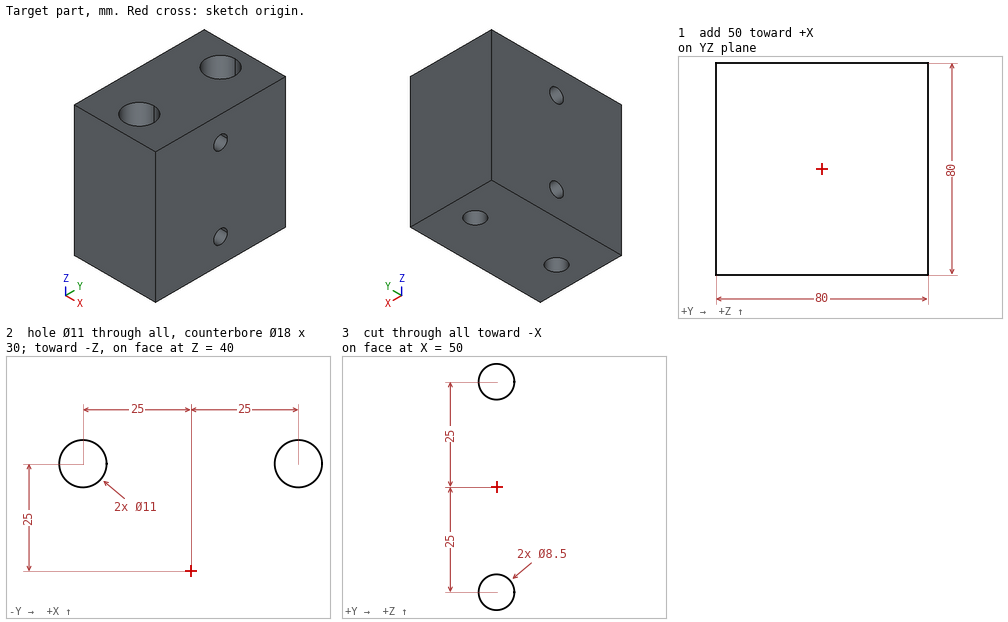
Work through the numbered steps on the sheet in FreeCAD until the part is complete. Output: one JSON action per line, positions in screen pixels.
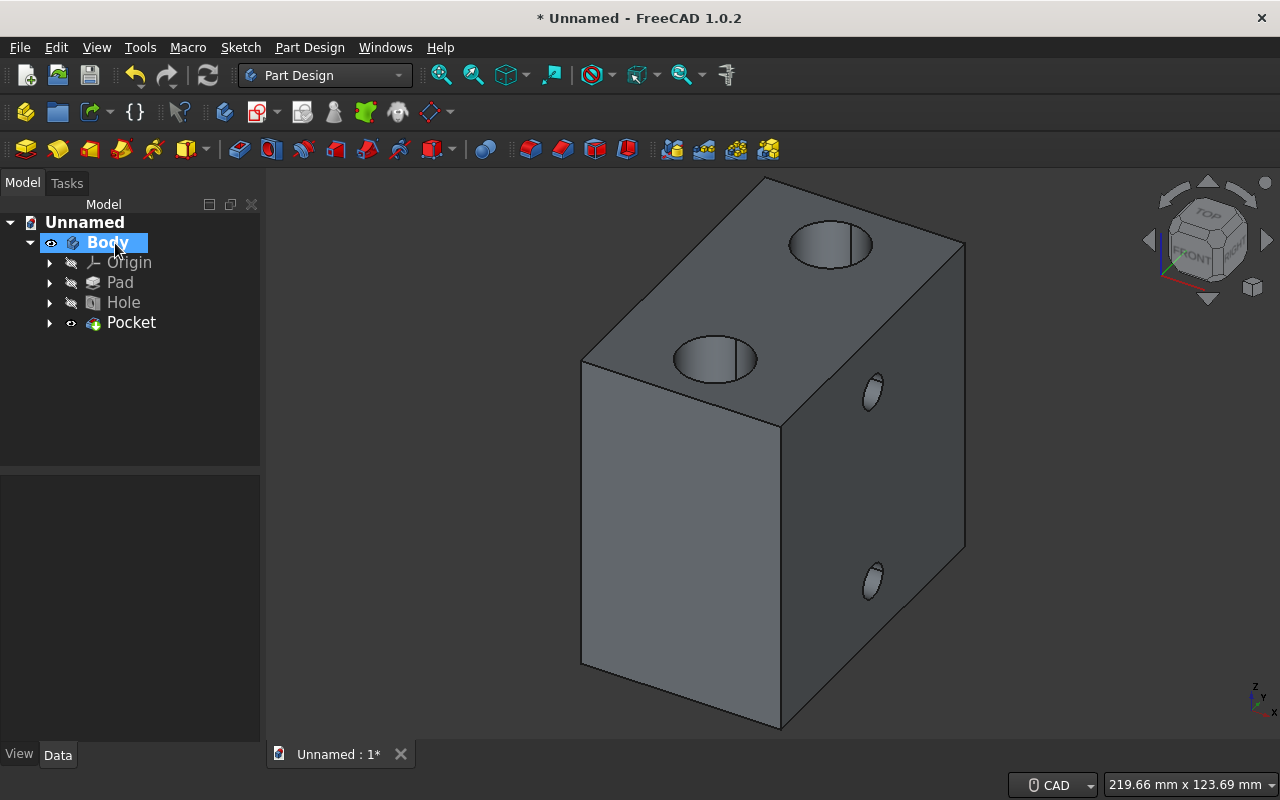
{"action": "key", "text": "0"}